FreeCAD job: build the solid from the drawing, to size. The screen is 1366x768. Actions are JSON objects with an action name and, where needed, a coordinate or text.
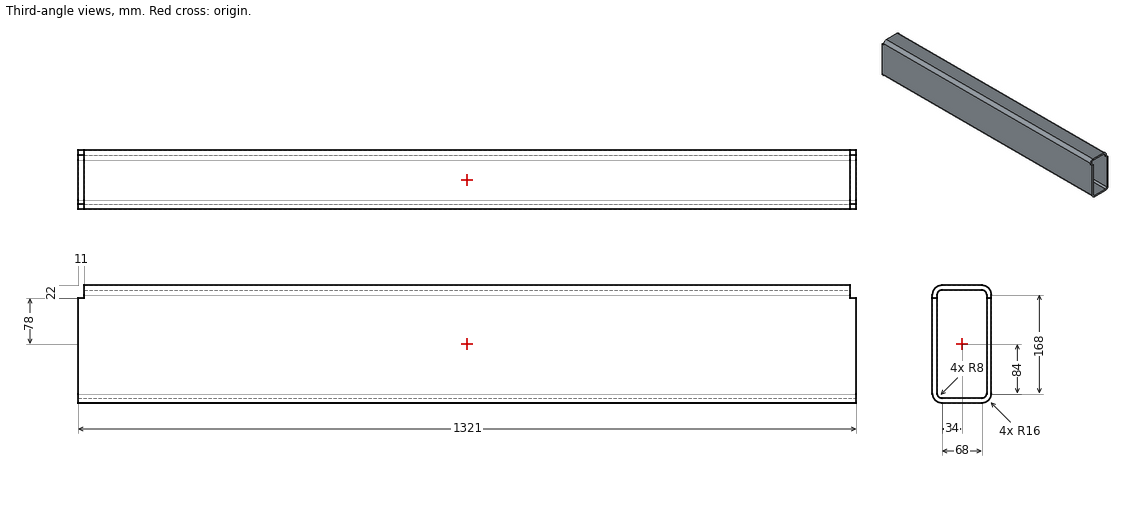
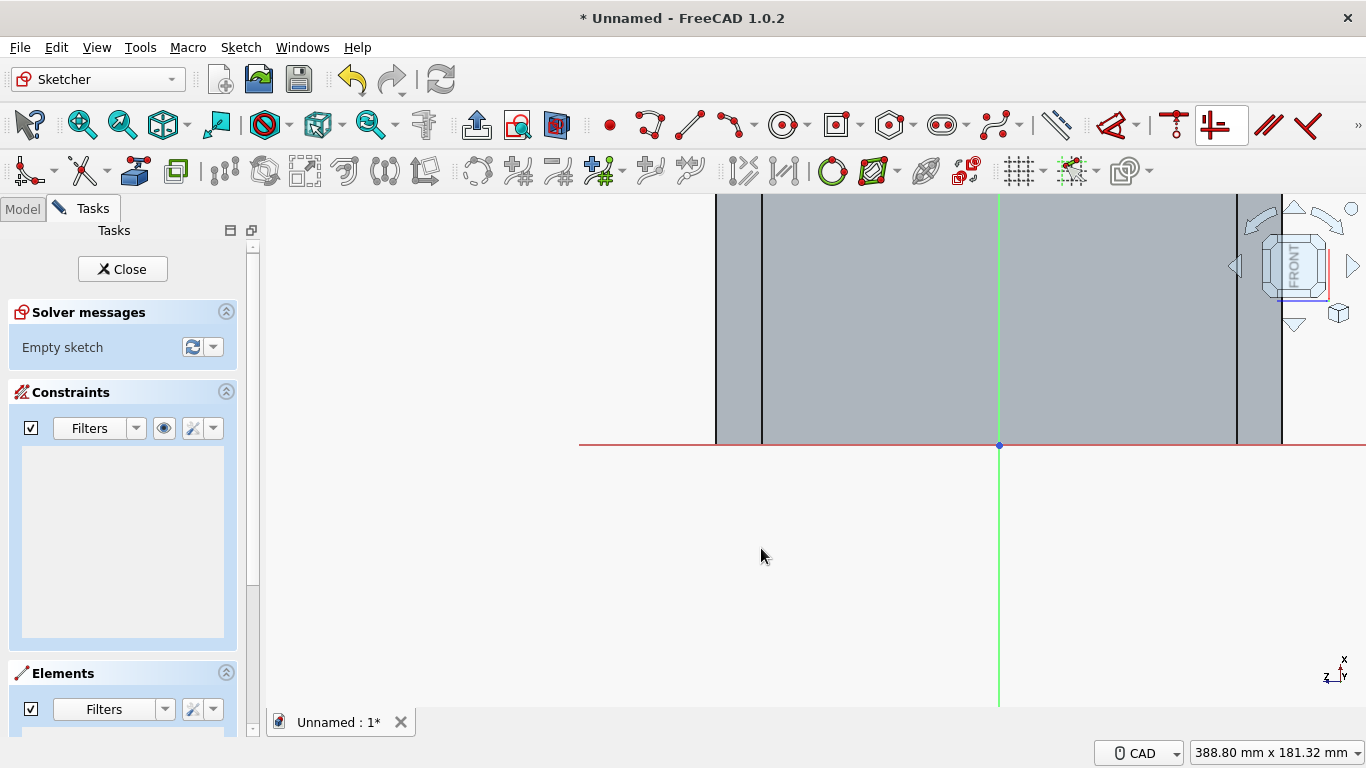
{"action": "scroll", "coordinate": [748, 428], "scroll_direction": "up", "scroll_amount": 12}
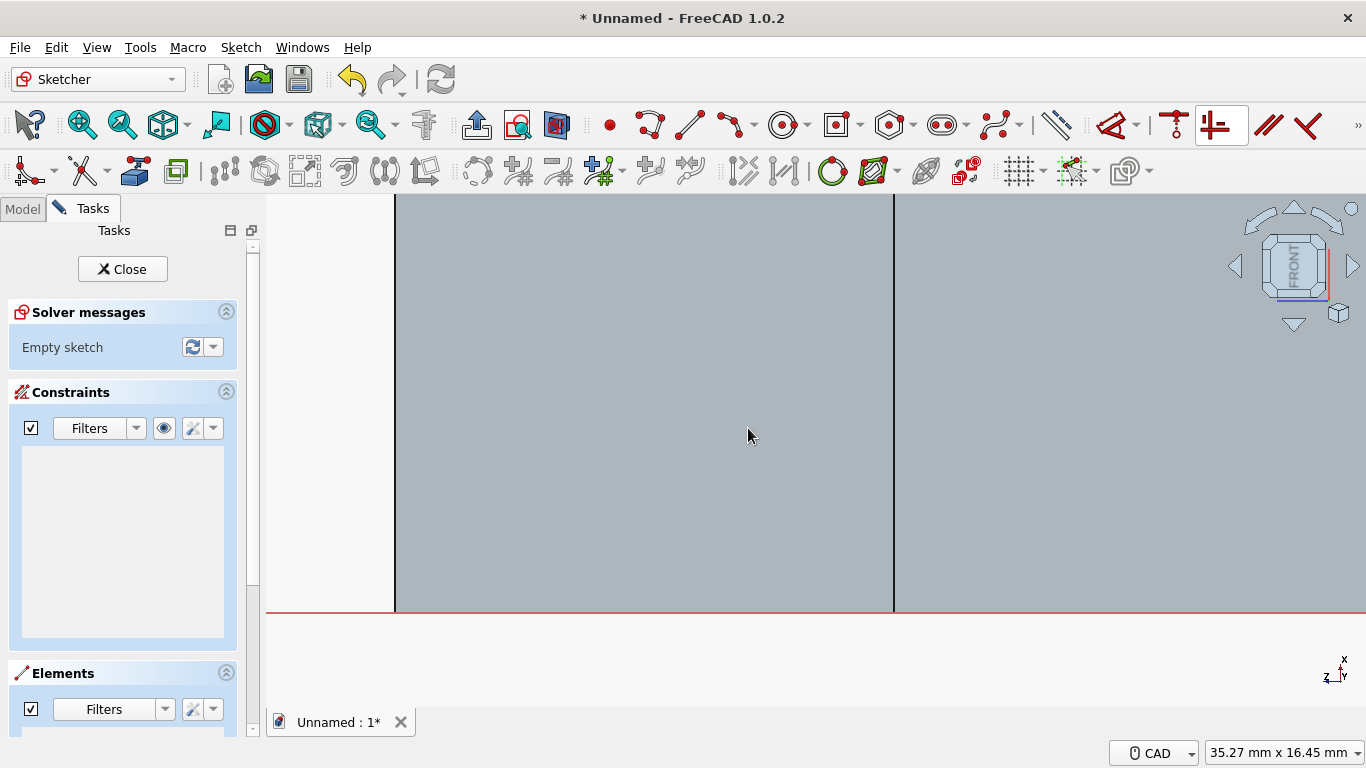
{"action": "key", "text": "g r"}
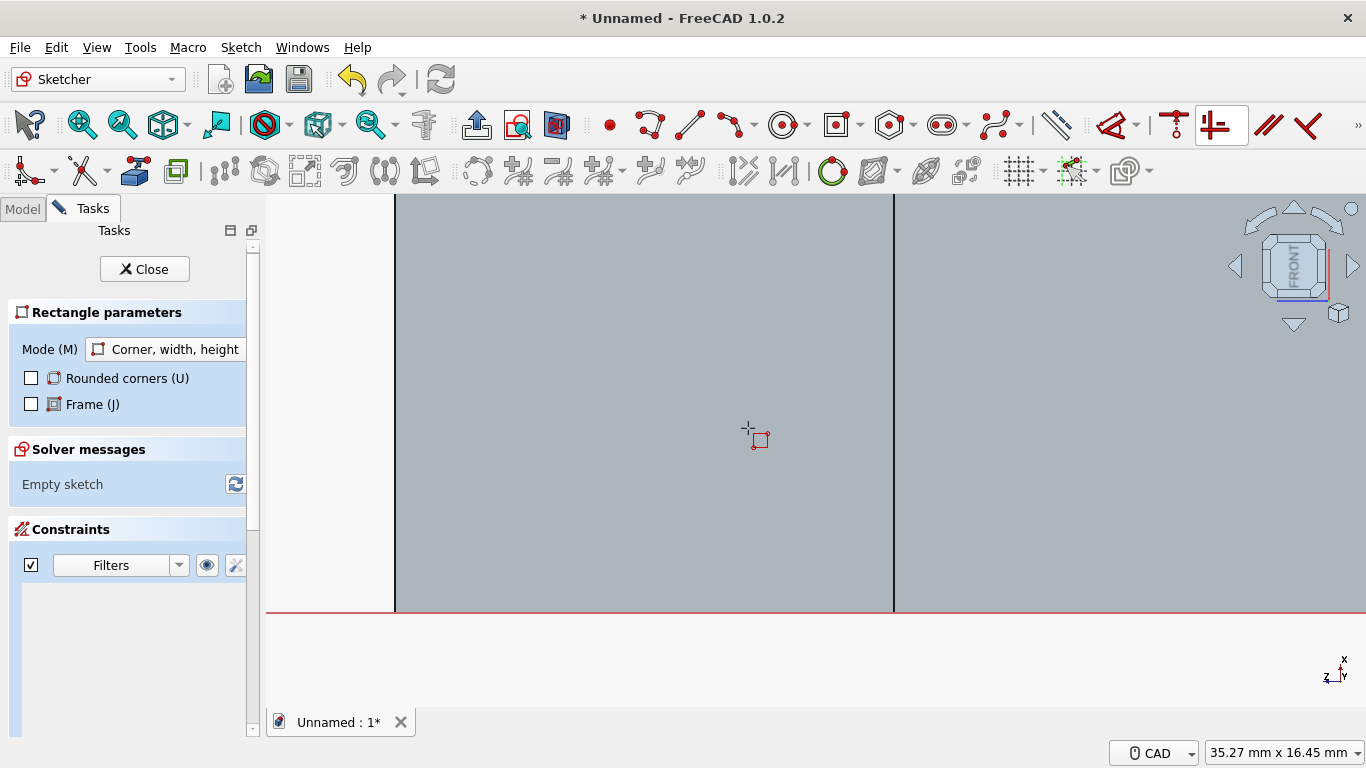
{"action": "left_click", "coordinate": [395, 270]}
{"action": "left_click", "coordinate": [1081, 613]}
{"action": "key", "text": "Escape"}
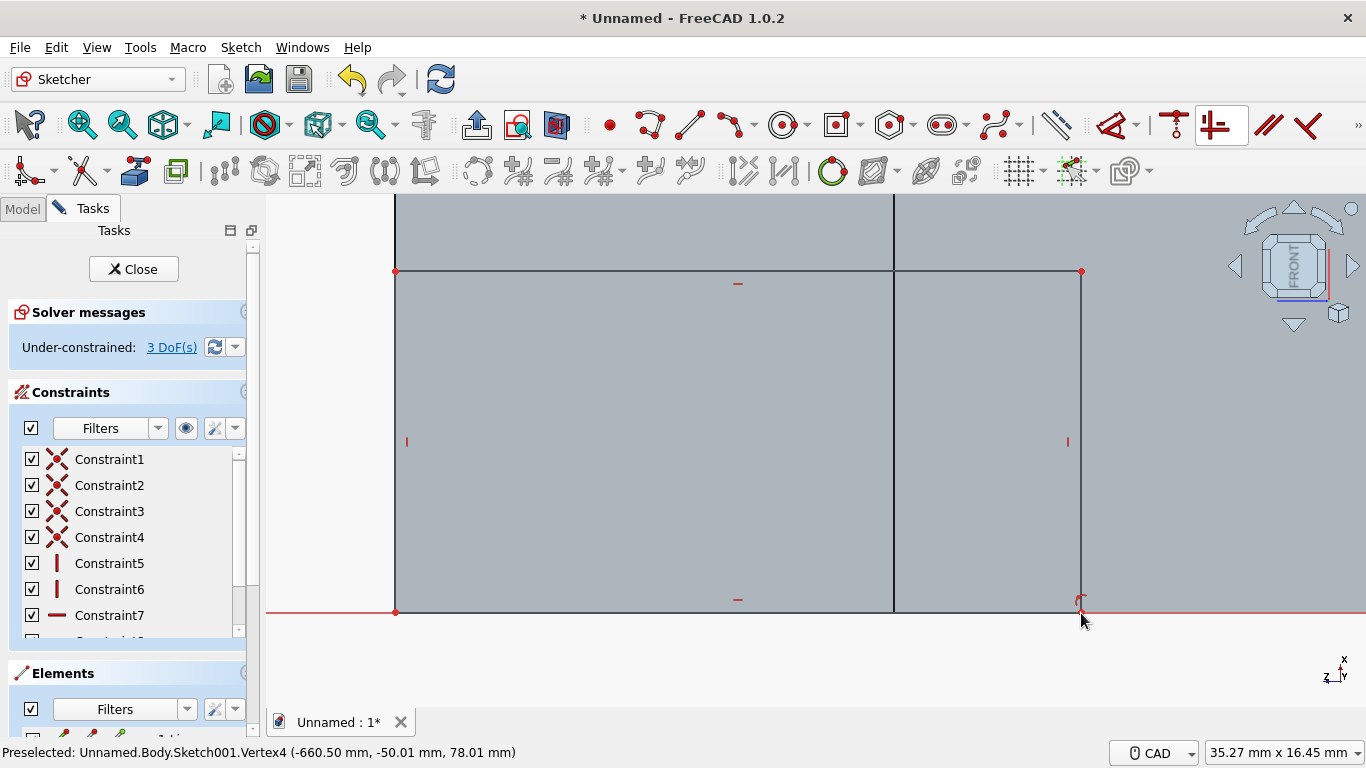
{"action": "key", "text": "d"}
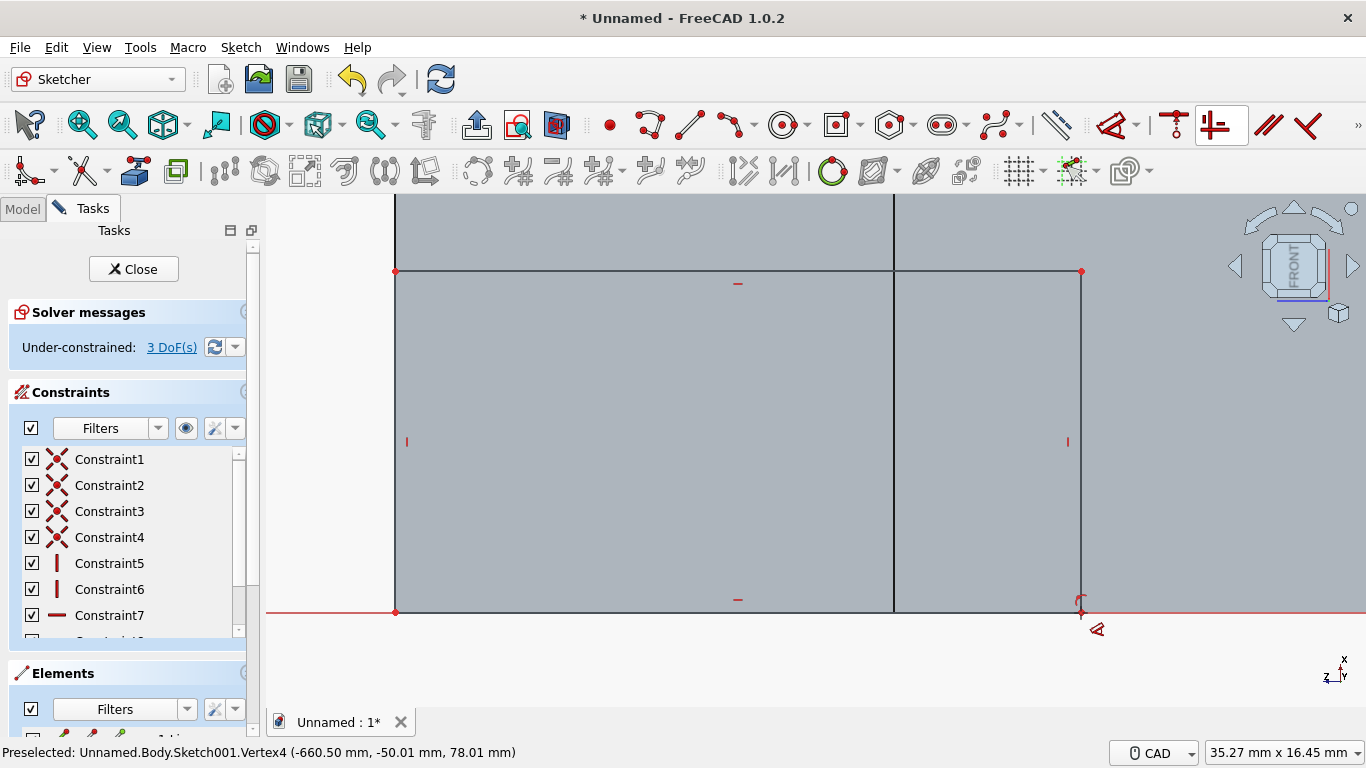
{"action": "left_click", "coordinate": [395, 374]}
{"action": "left_click", "coordinate": [361, 442]}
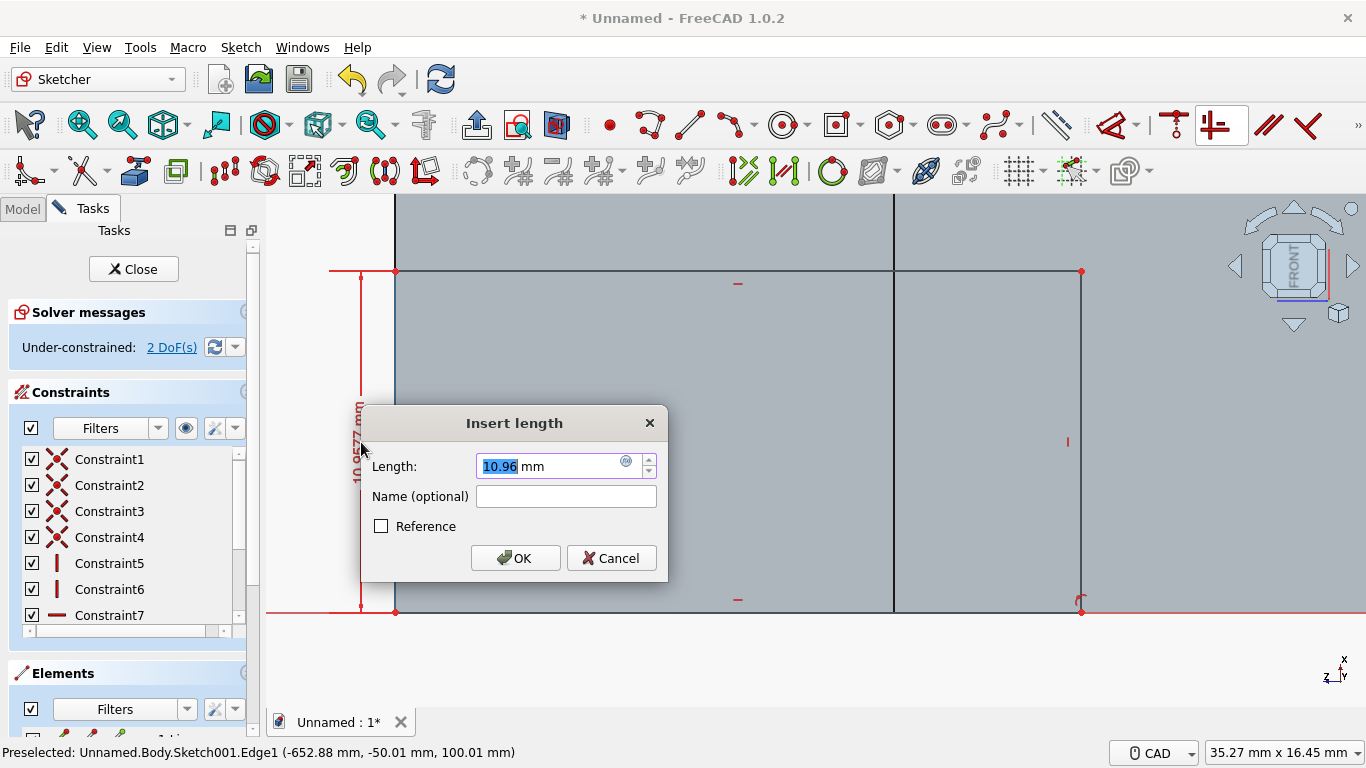
{"action": "type", "text": "11"}
{"action": "key", "text": "Return"}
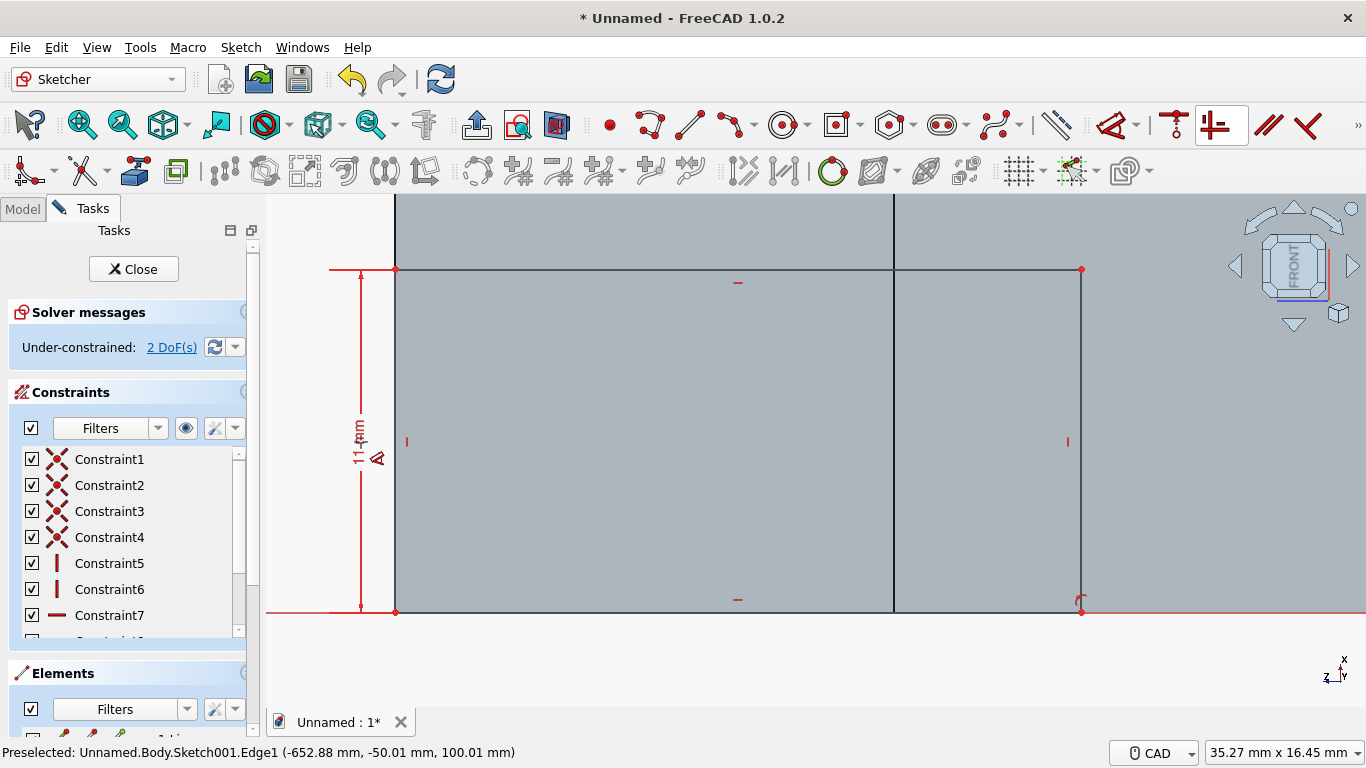
{"action": "left_click", "coordinate": [601, 613]}
{"action": "left_click", "coordinate": [738, 647]}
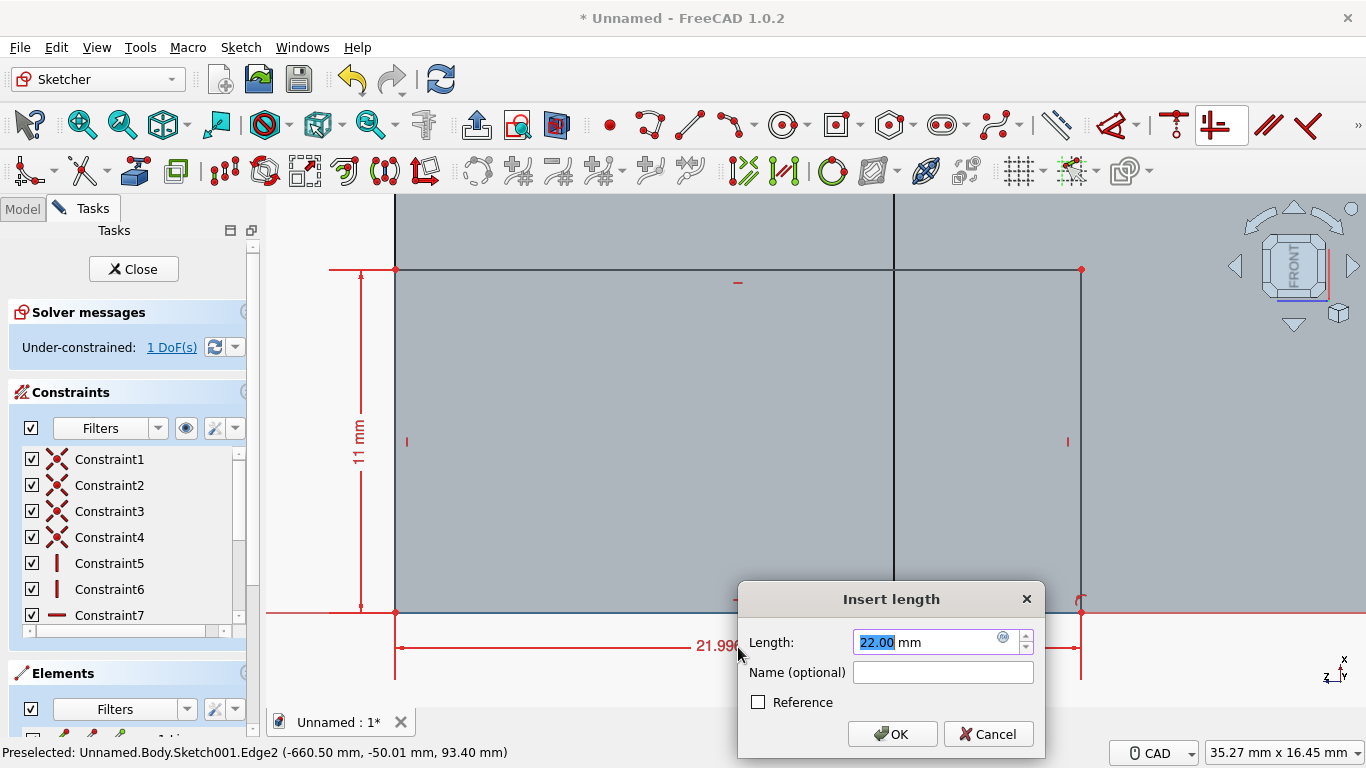
{"action": "type", "text": "22"}
{"action": "key", "text": "Return"}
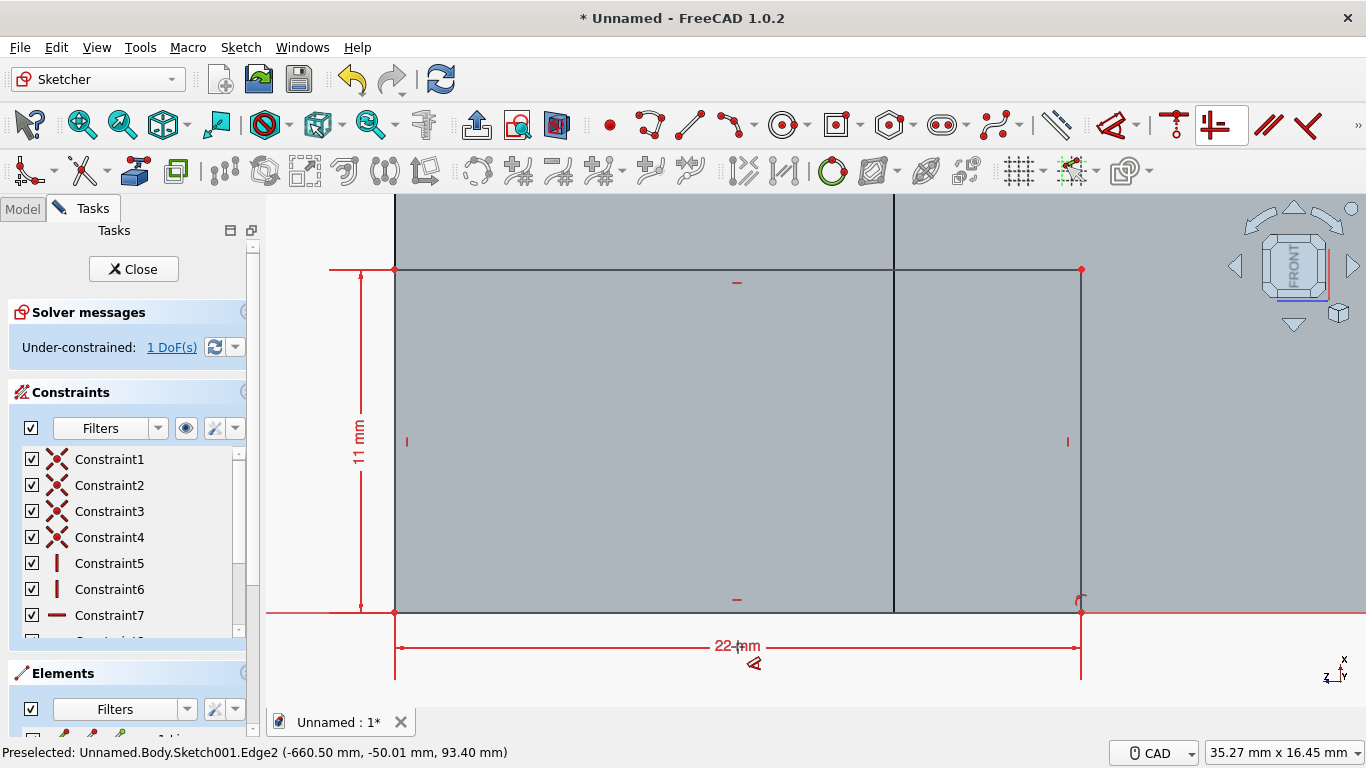
{"action": "left_click", "coordinate": [1081, 613]}
{"action": "left_click", "coordinate": [1141, 647]}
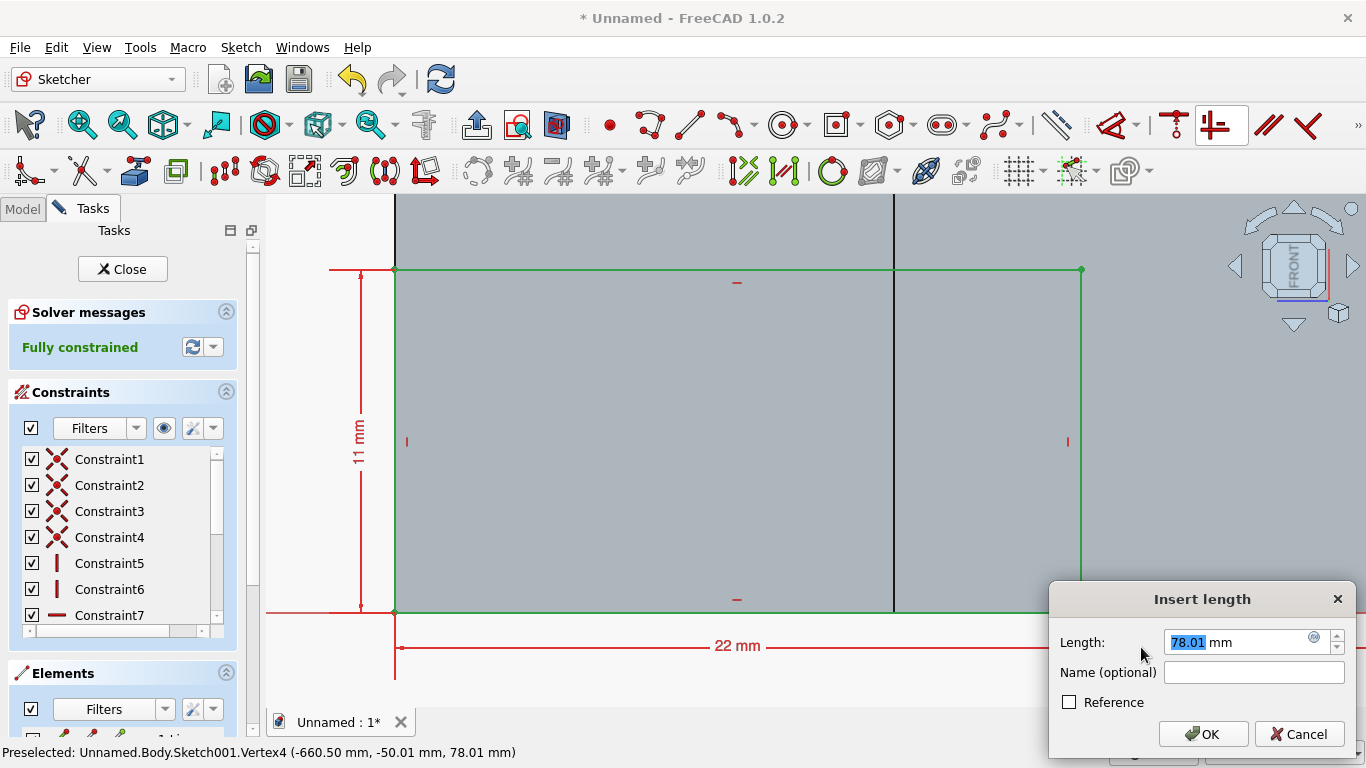
{"action": "type", "text": "78"}
{"action": "key", "text": "Return"}
{"action": "key", "text": "Escape"}